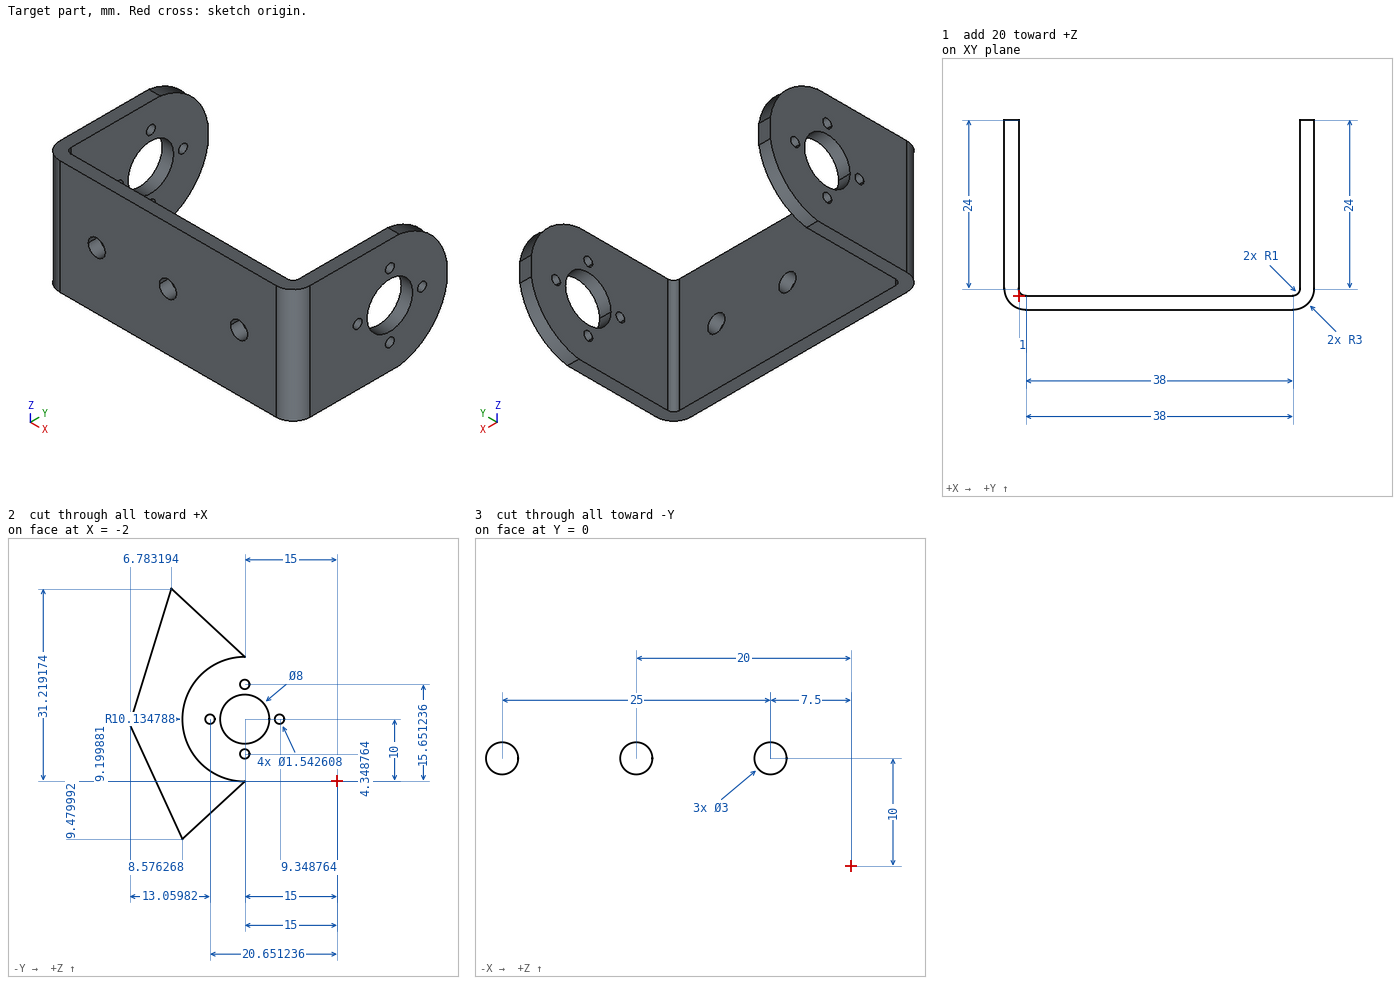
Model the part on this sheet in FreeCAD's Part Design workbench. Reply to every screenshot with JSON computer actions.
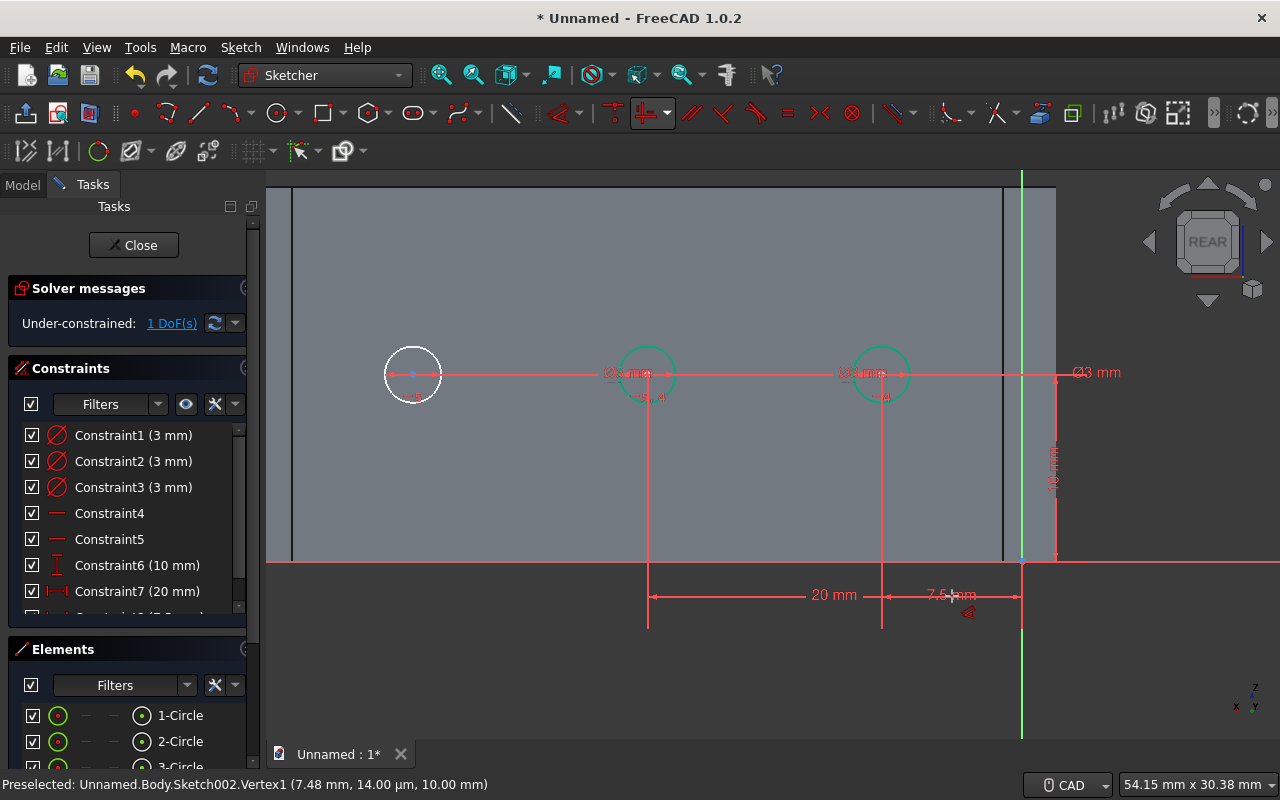
{"action": "left_click", "coordinate": [882, 375]}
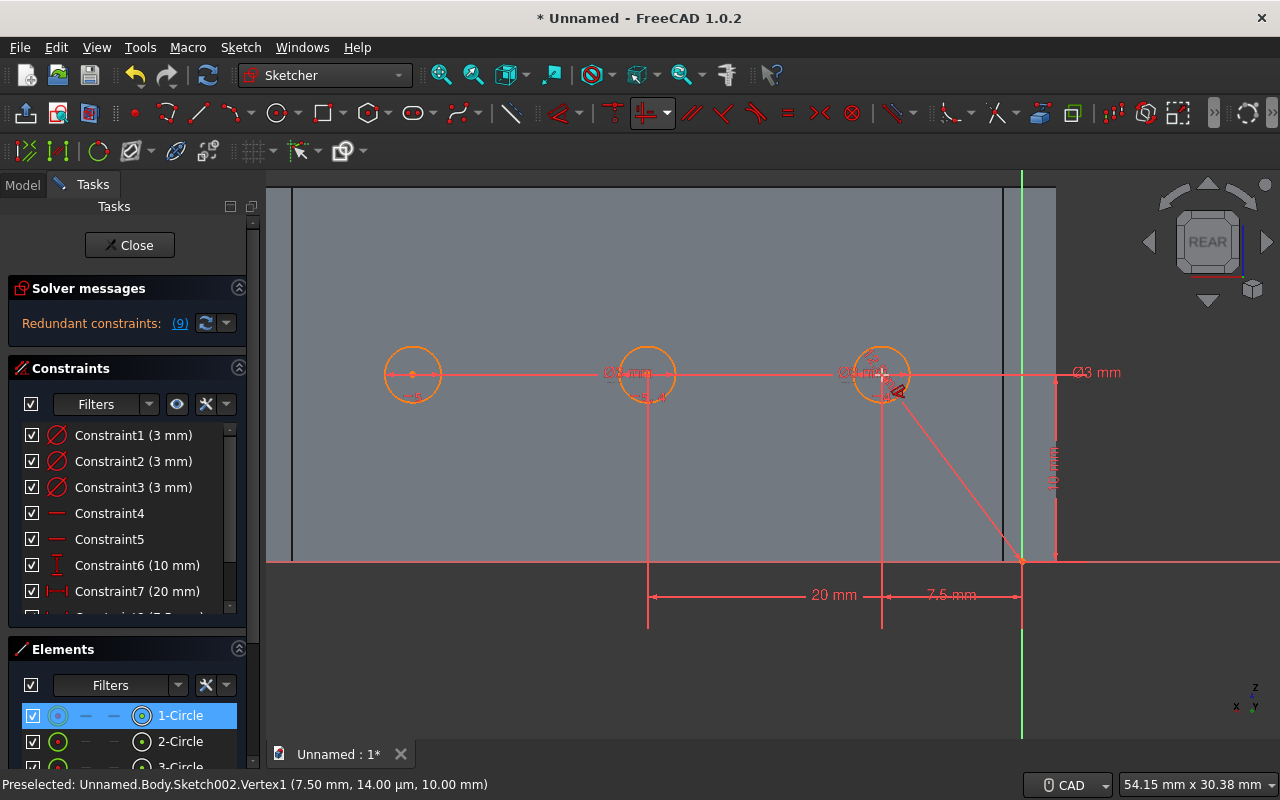
{"action": "left_click", "coordinate": [413, 375]}
{"action": "left_click", "coordinate": [540, 341]}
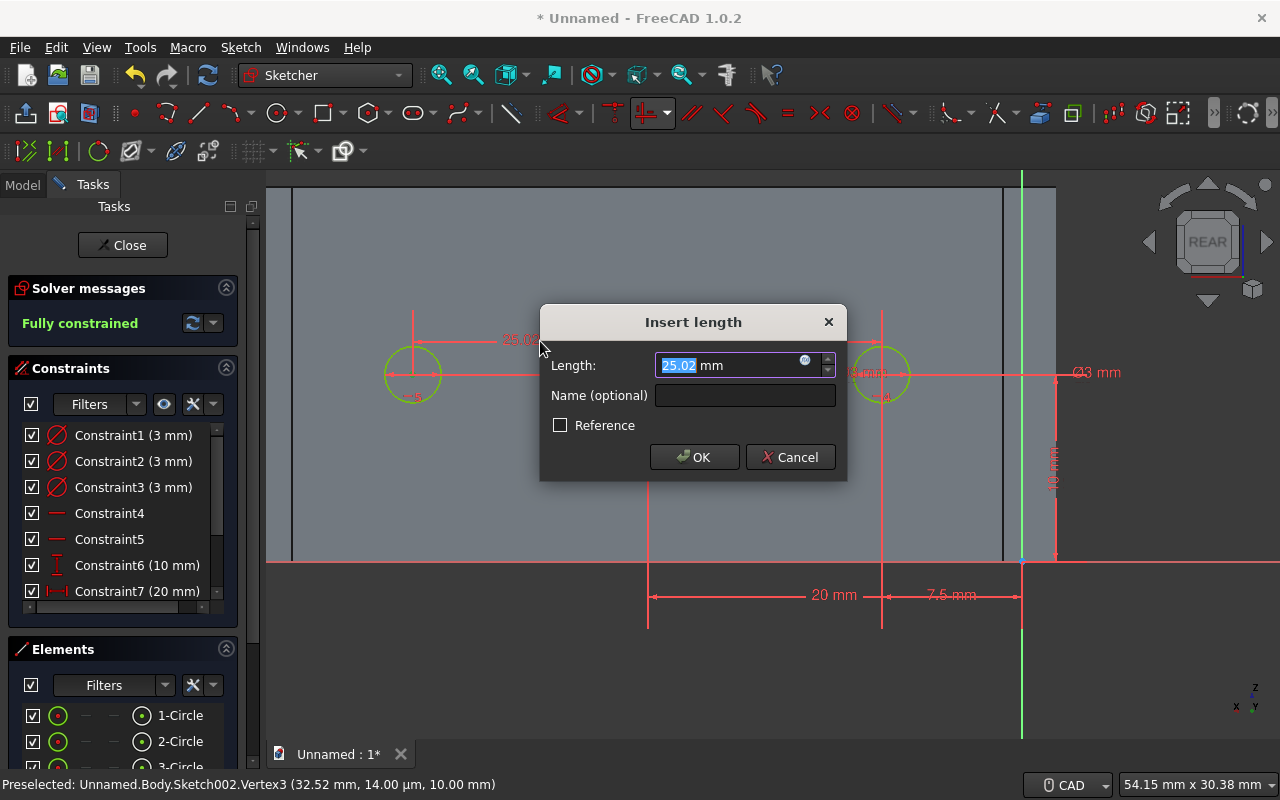
{"action": "type", "text": "25"}
{"action": "key", "text": "Return"}
{"action": "key", "text": "Escape"}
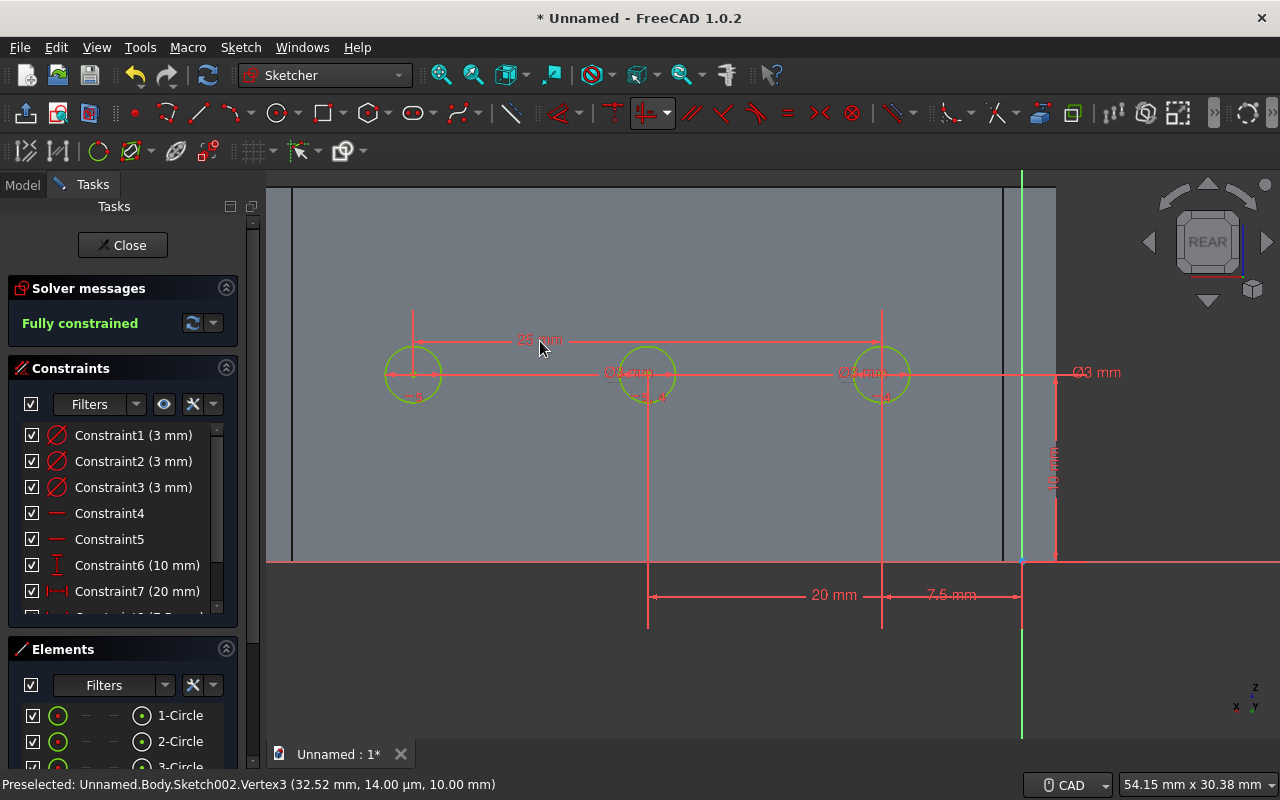
{"action": "left_click", "coordinate": [123, 245]}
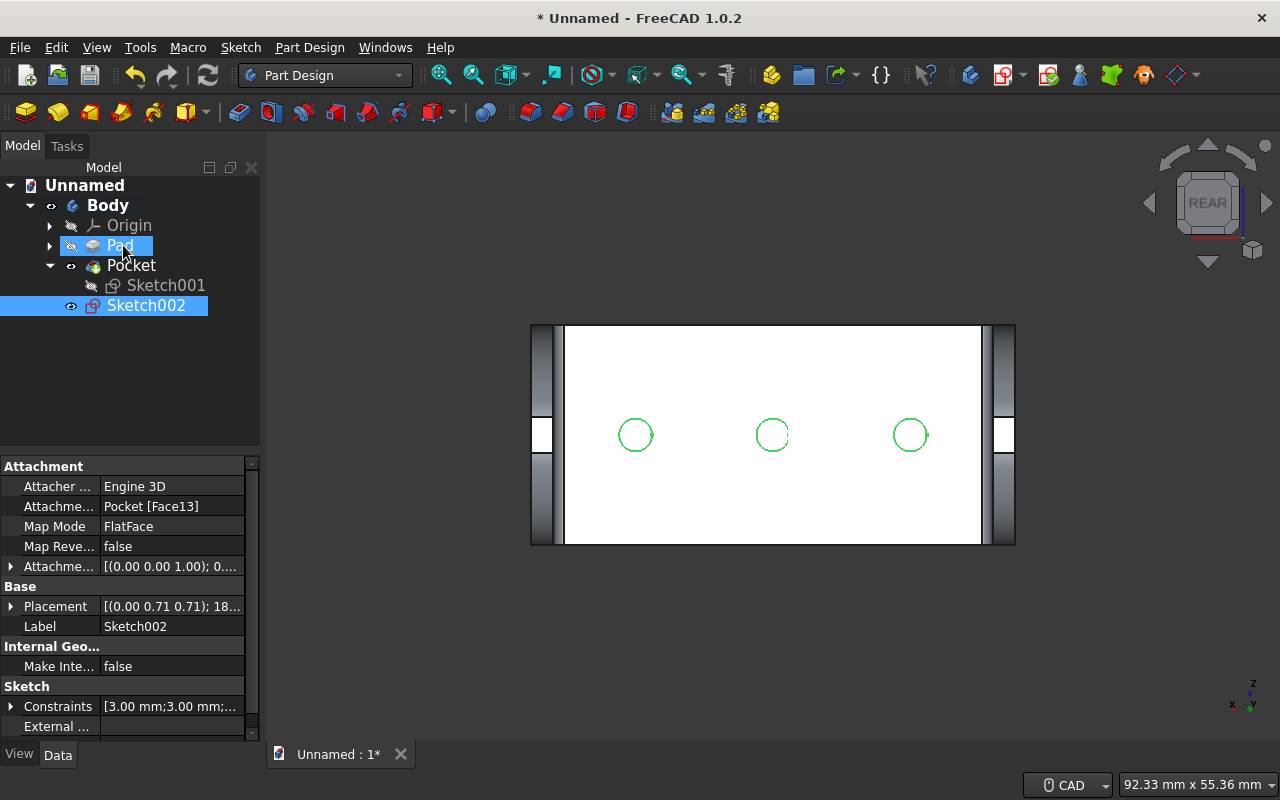
{"action": "left_click", "coordinate": [240, 112]}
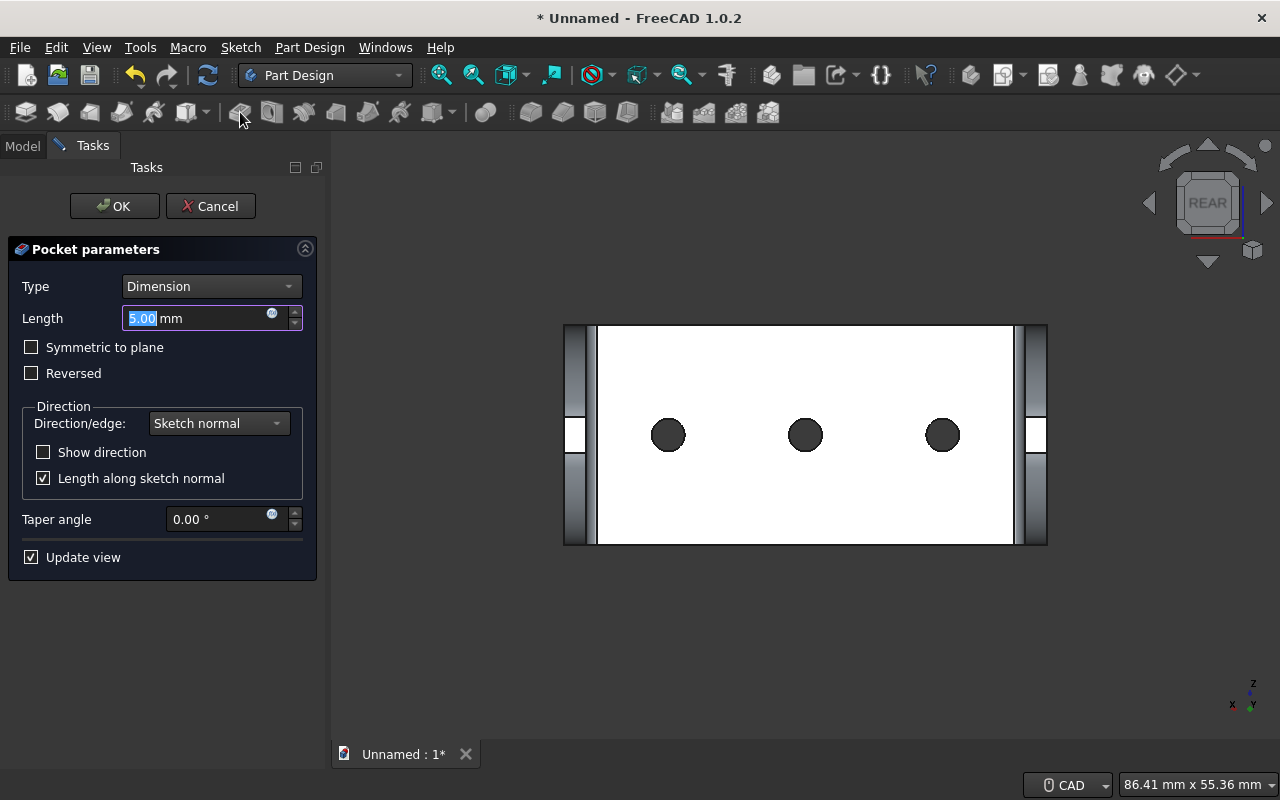
{"action": "left_click", "coordinate": [212, 286]}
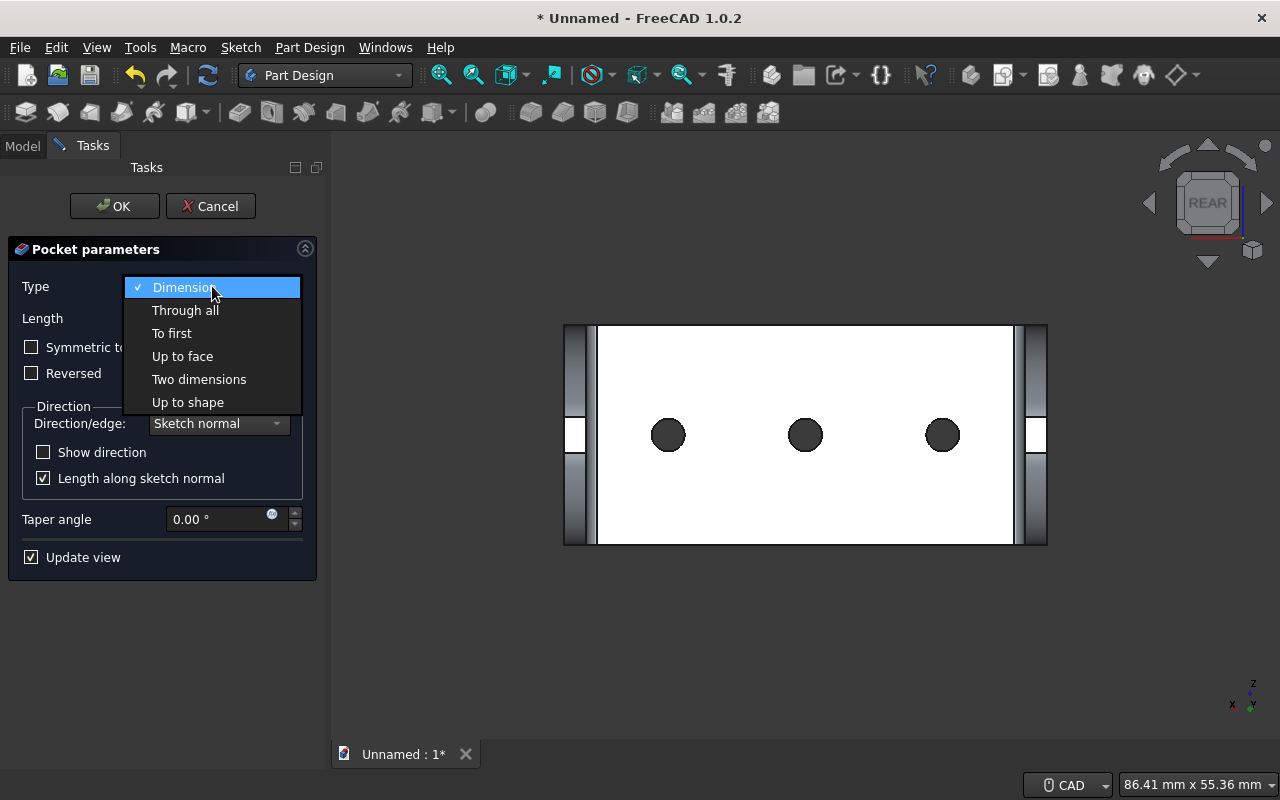
{"action": "left_click", "coordinate": [212, 310]}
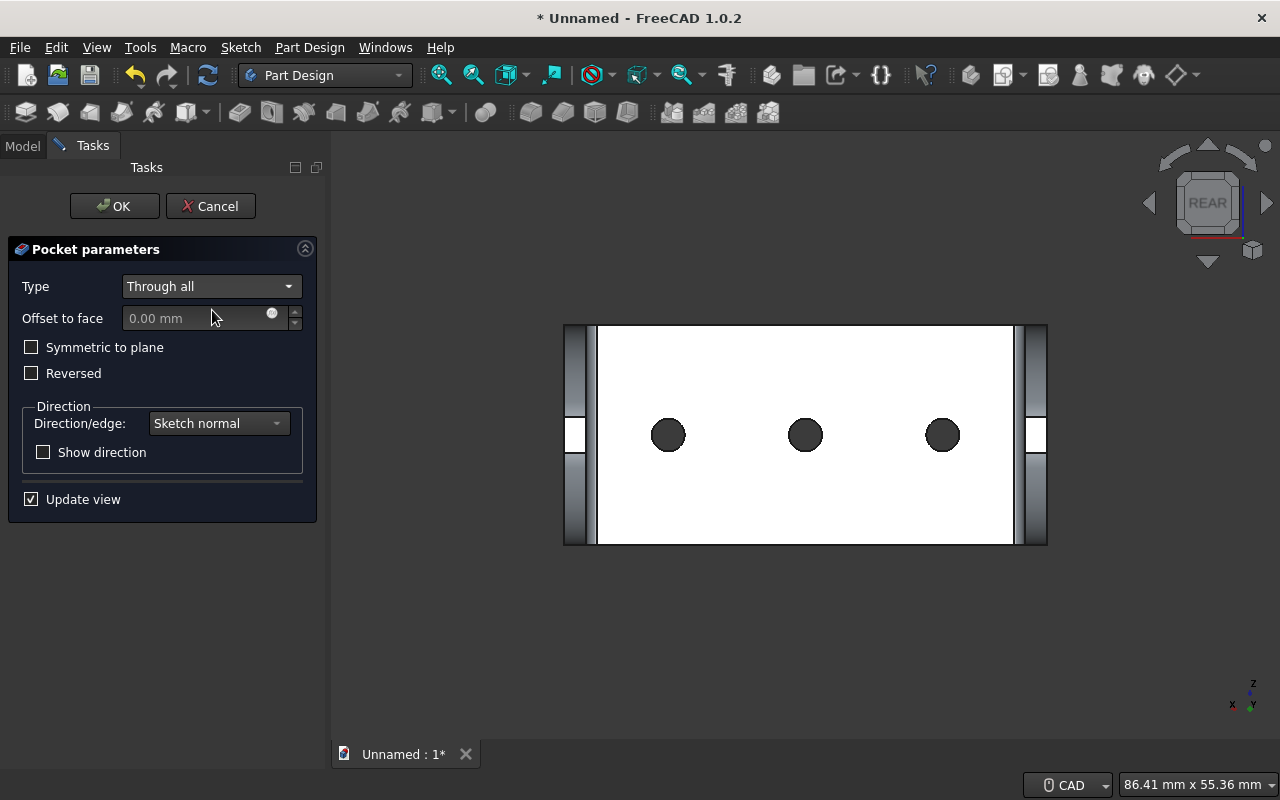
{"action": "left_click", "coordinate": [115, 206]}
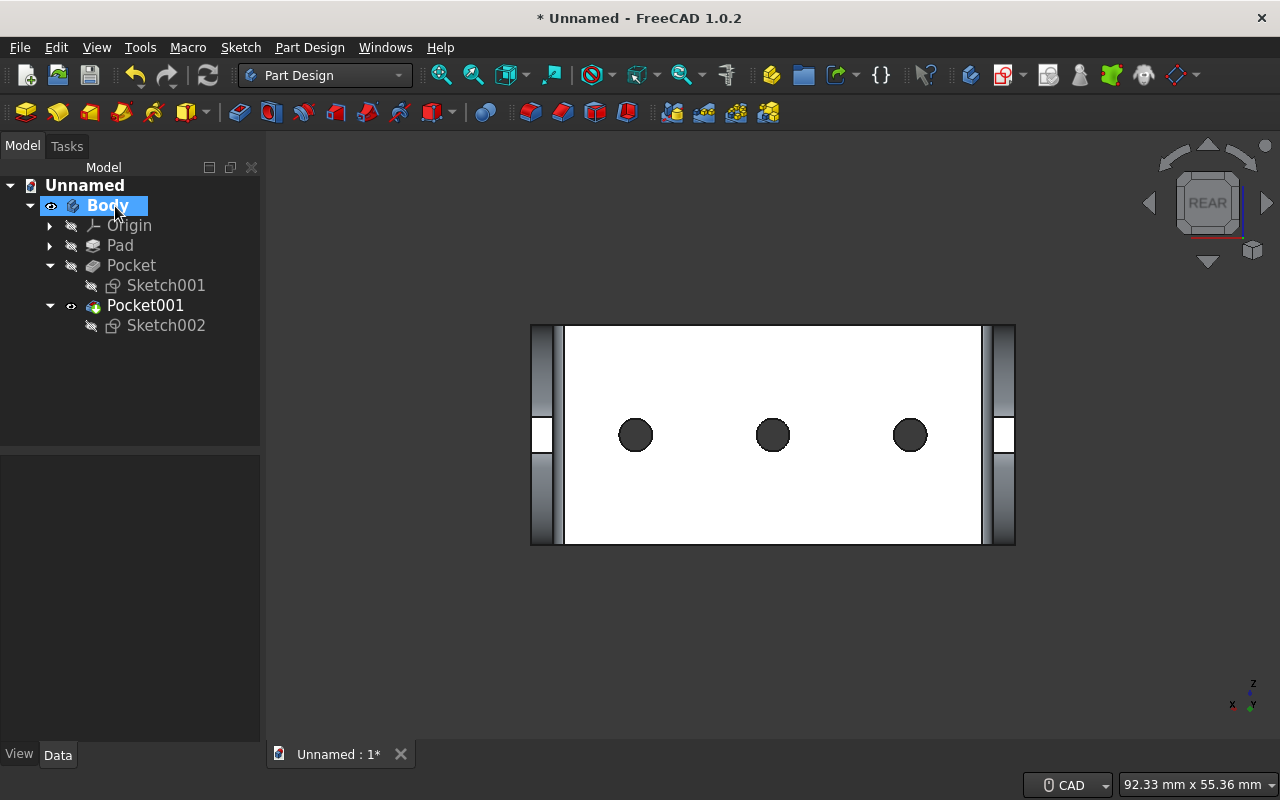
{"action": "key", "text": "0"}